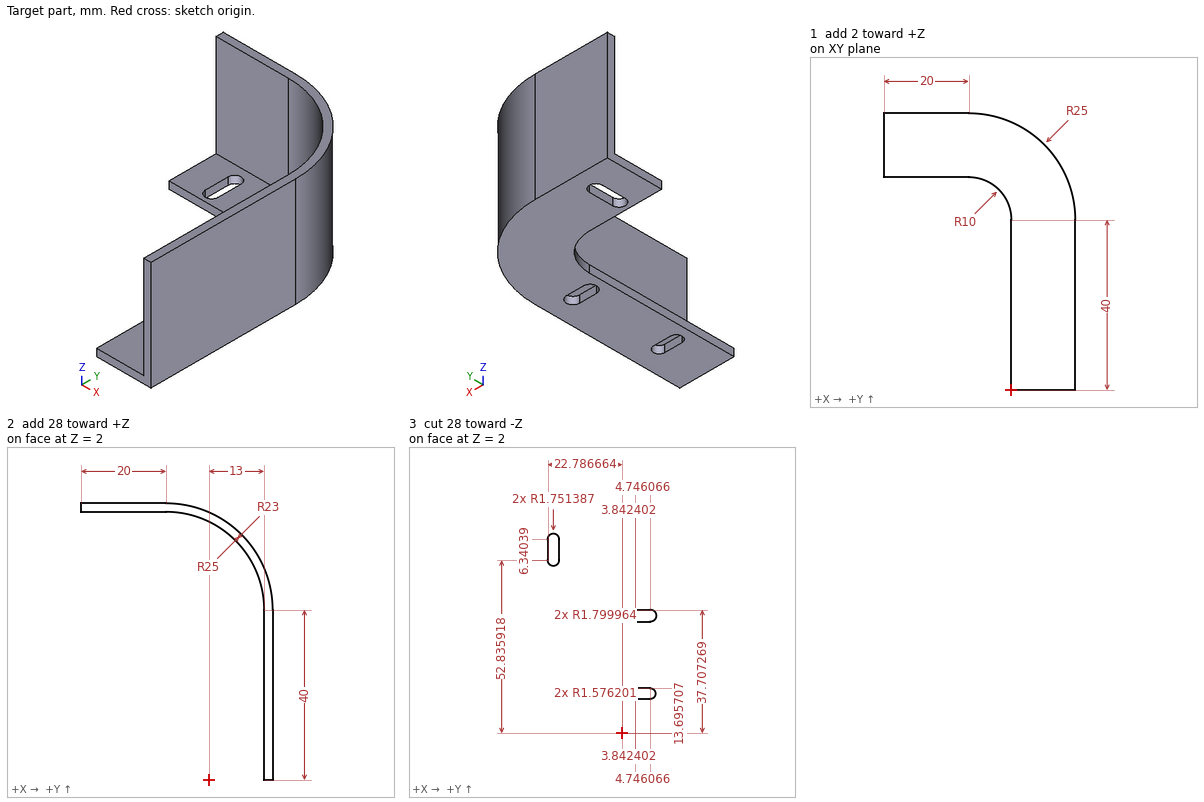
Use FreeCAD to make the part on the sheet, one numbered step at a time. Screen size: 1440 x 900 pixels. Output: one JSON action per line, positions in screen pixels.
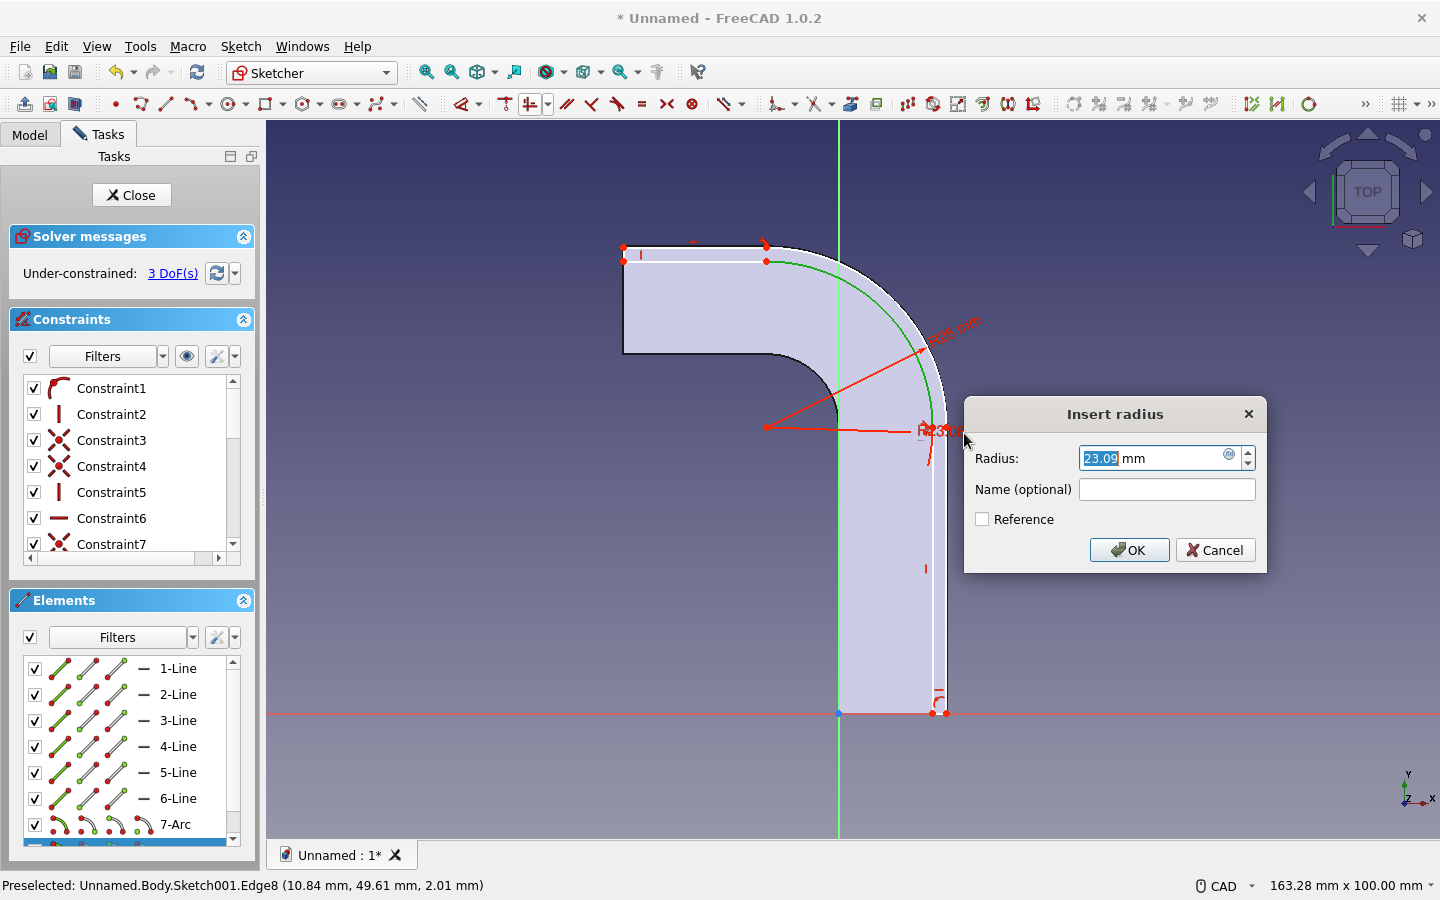
{"action": "type", "text": "23"}
{"action": "key", "text": "Return"}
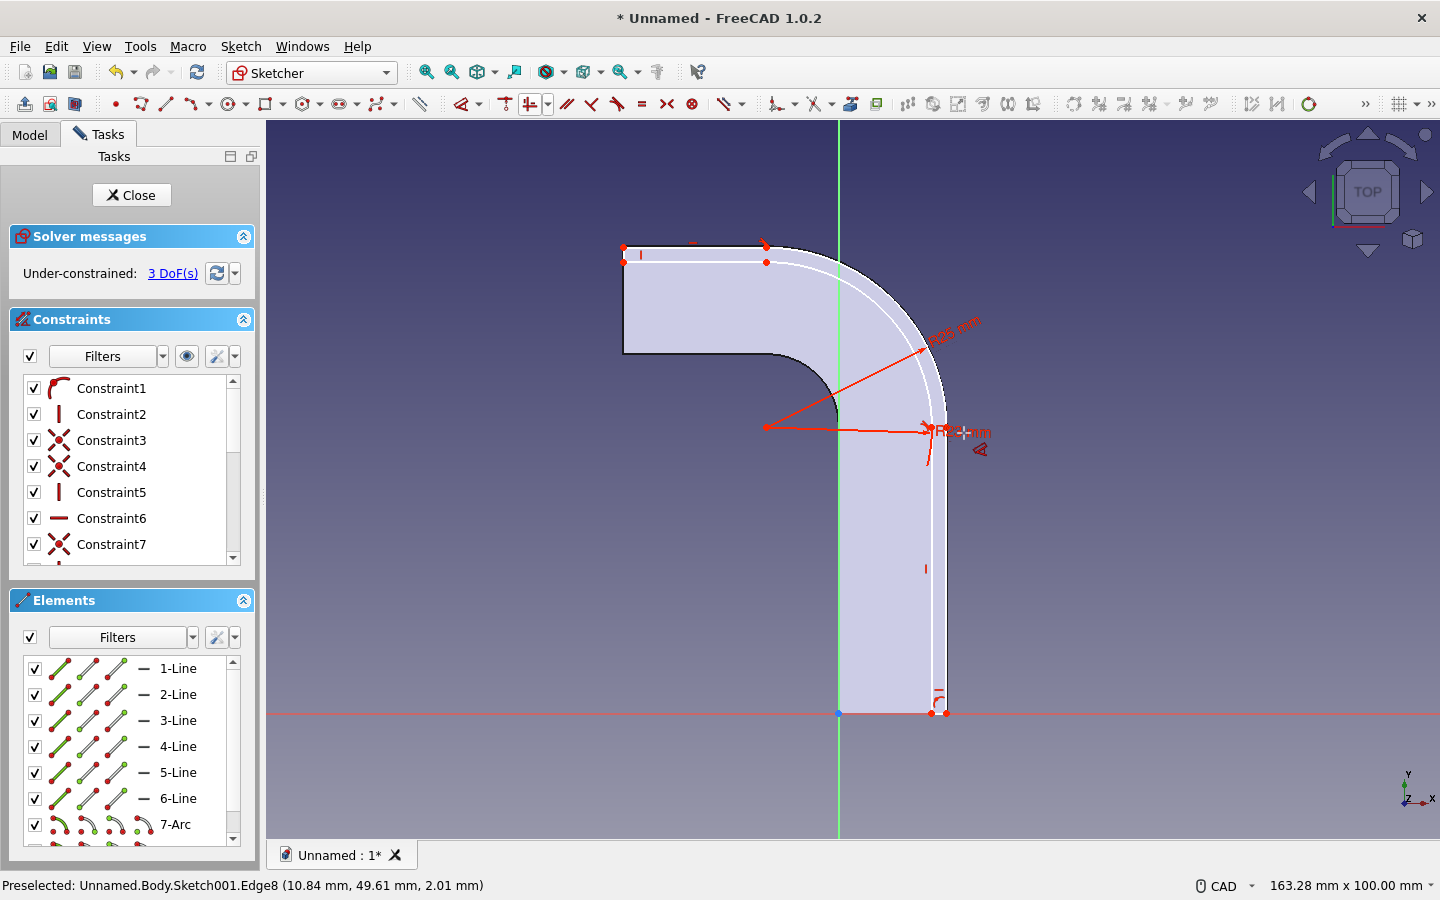
{"action": "left_click", "coordinate": [932, 513]}
{"action": "left_click", "coordinate": [966, 571]}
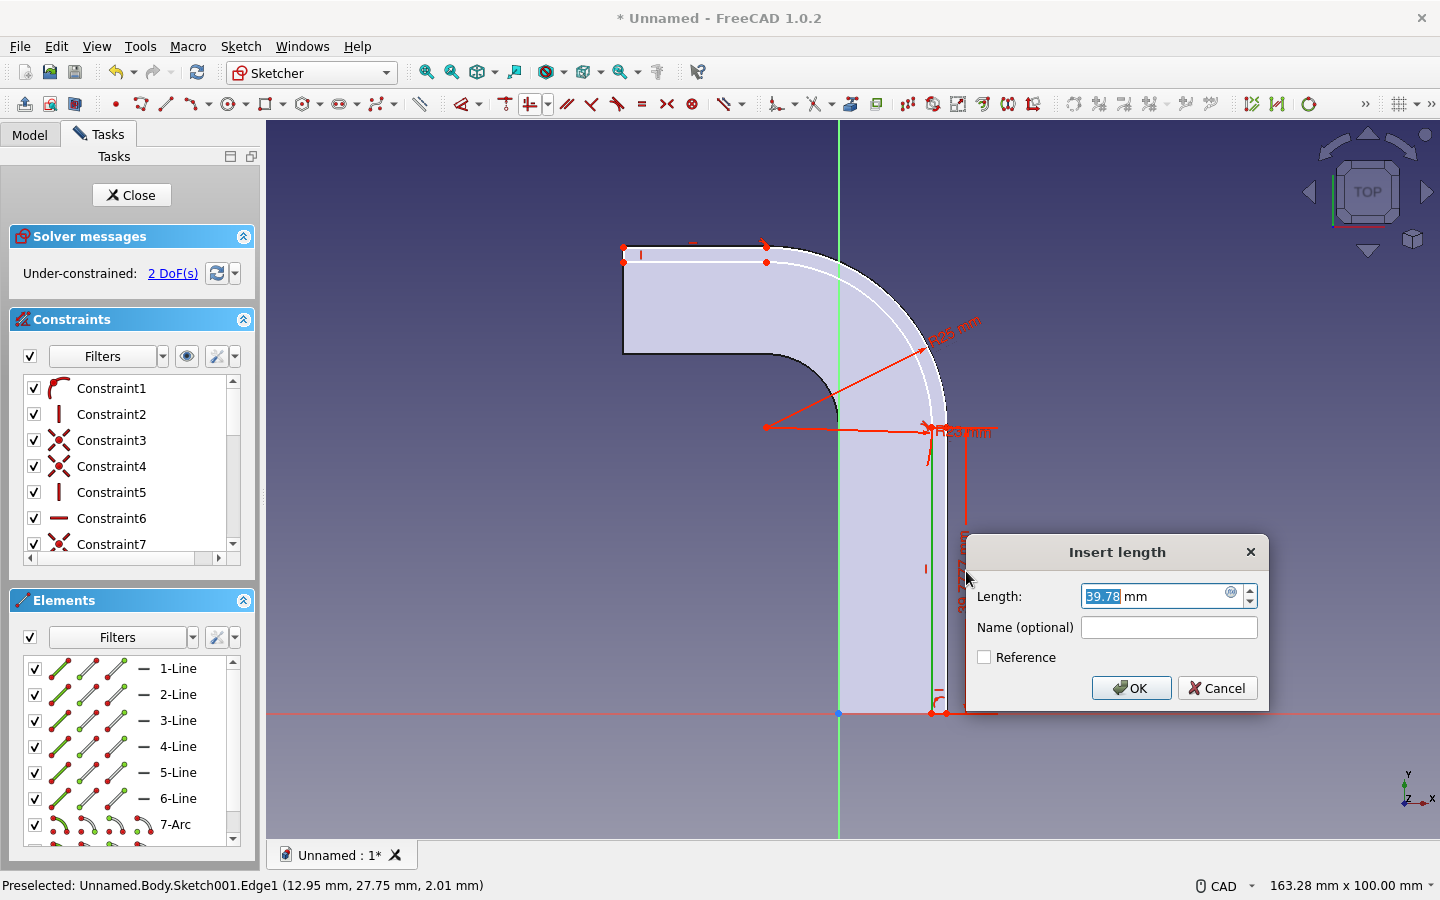
{"action": "type", "text": "40"}
{"action": "key", "text": "Return"}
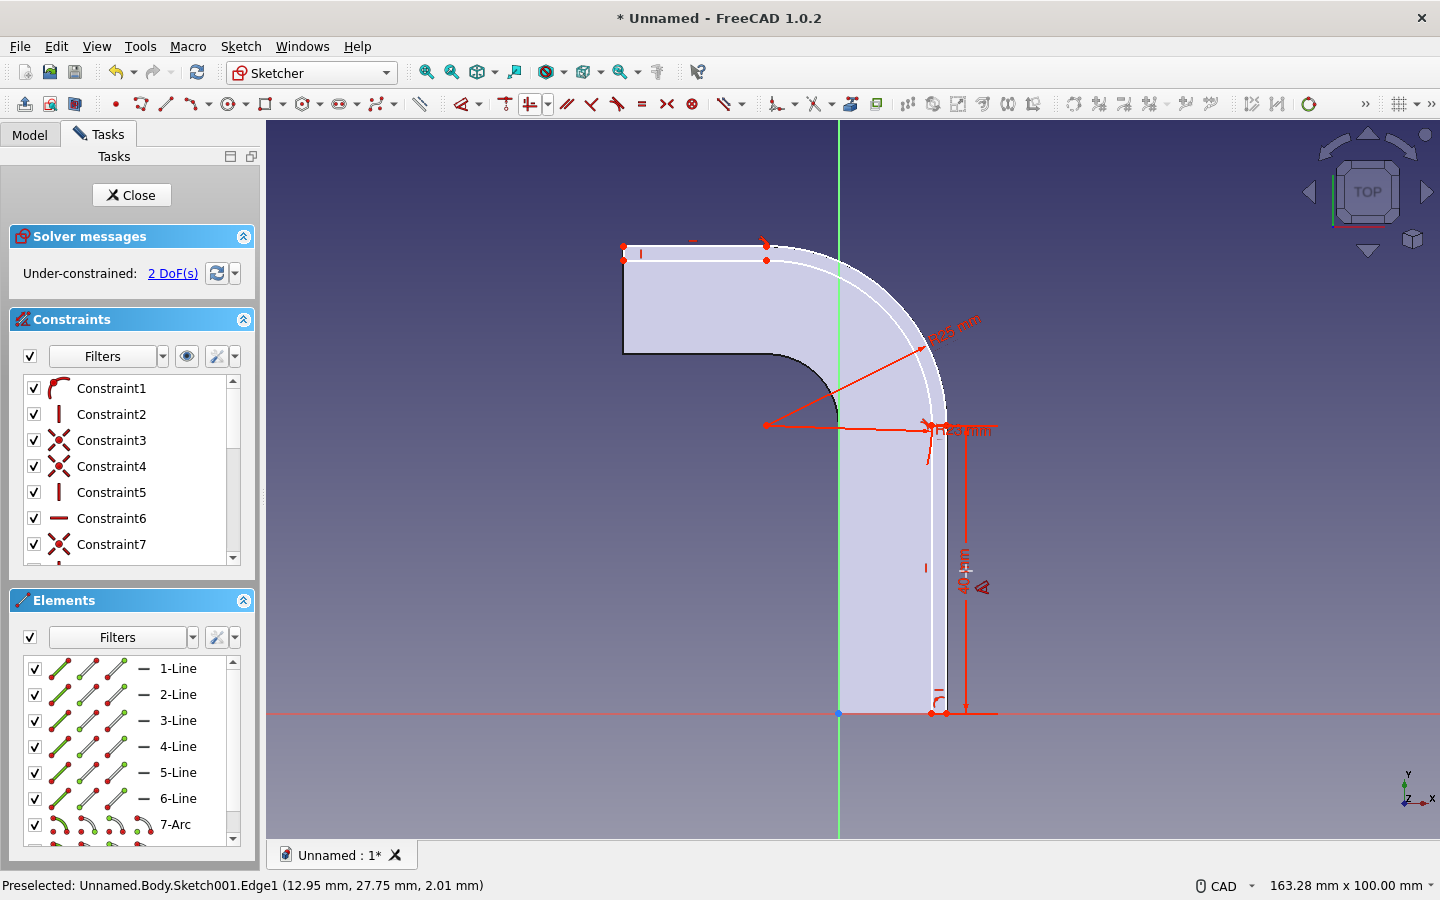
{"action": "left_click", "coordinate": [724, 246]}
{"action": "left_click", "coordinate": [695, 212]}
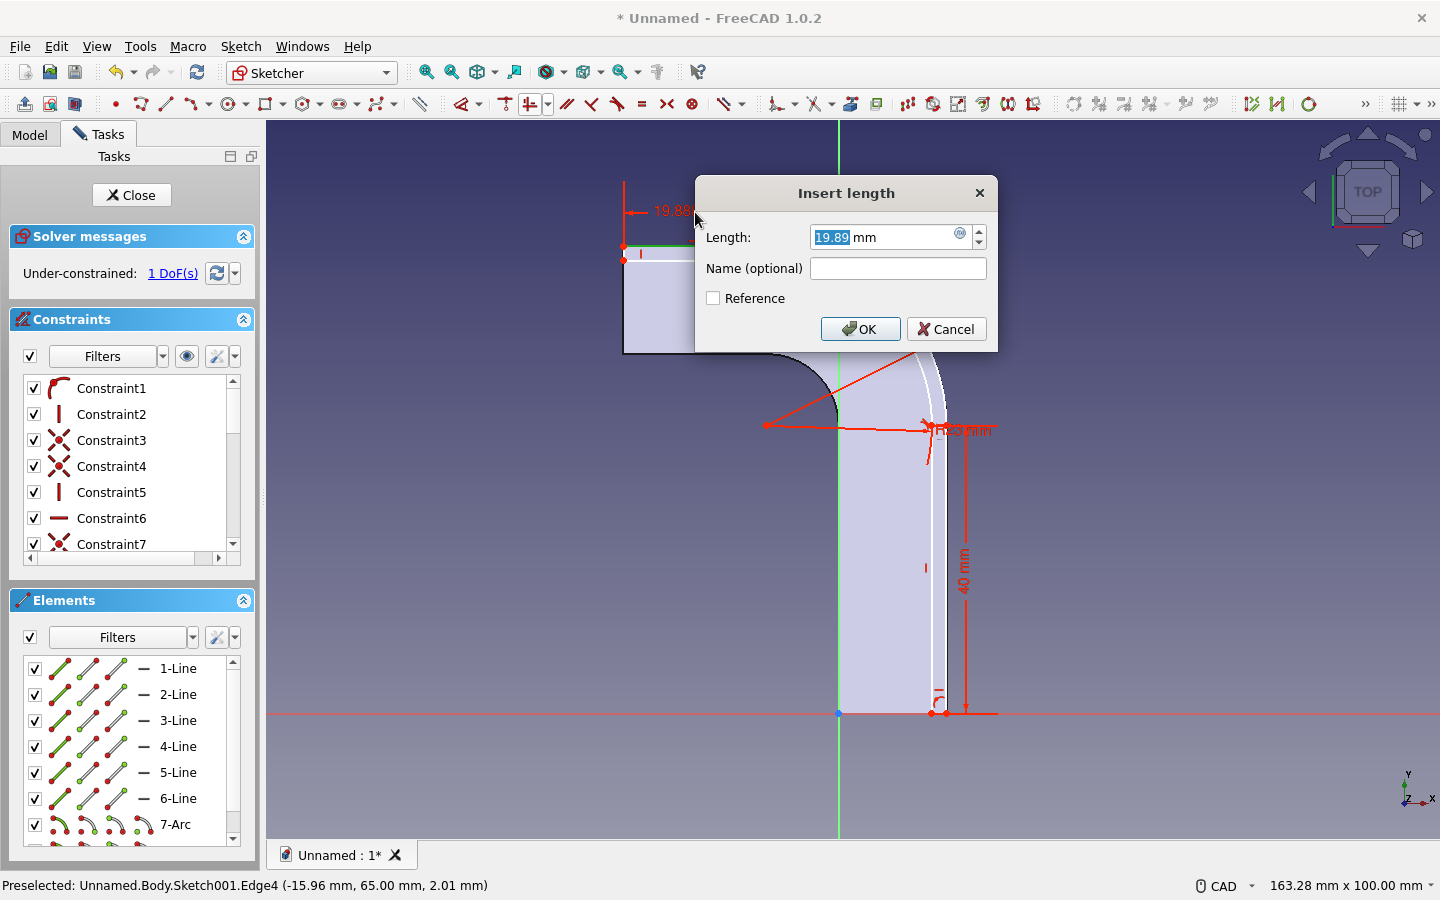
{"action": "type", "text": "20"}
{"action": "key", "text": "Return"}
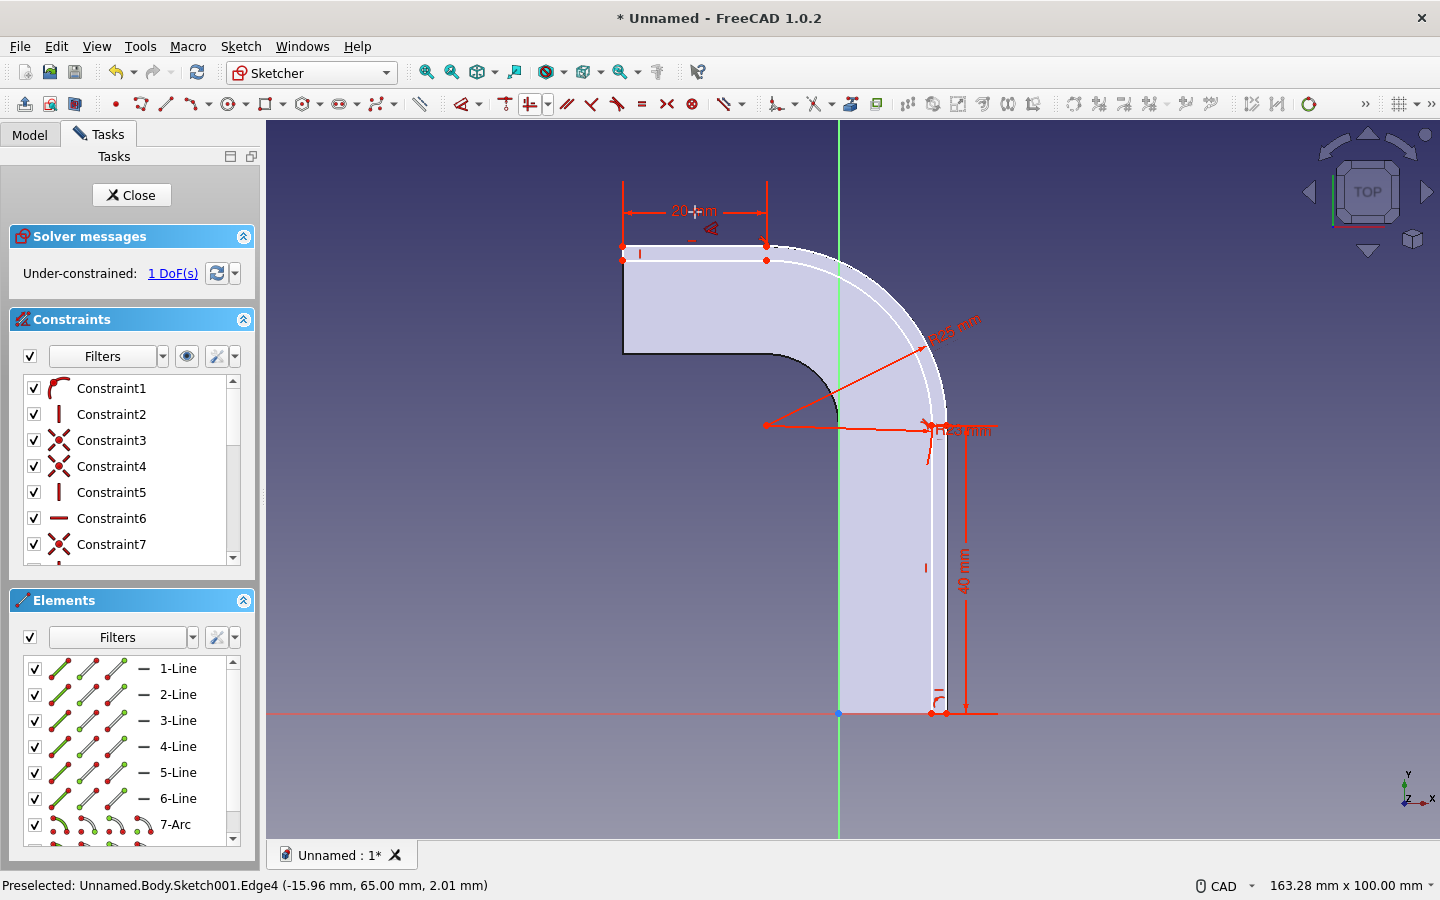
{"action": "left_click", "coordinate": [932, 426]}
{"action": "left_click", "coordinate": [885, 748]}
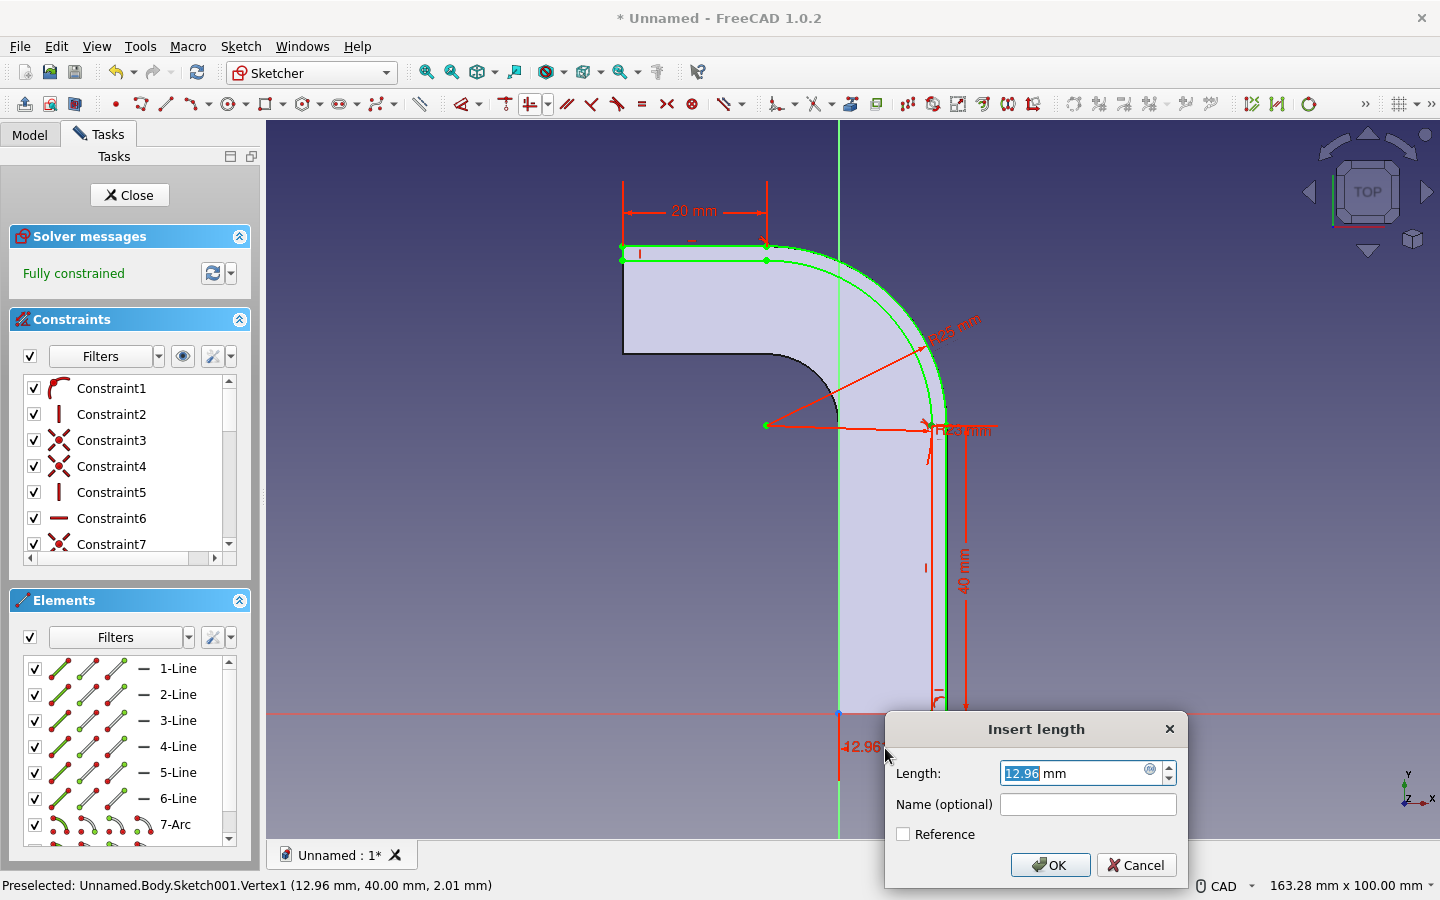
{"action": "type", "text": "13"}
{"action": "key", "text": "Return"}
{"action": "key", "text": "Escape"}